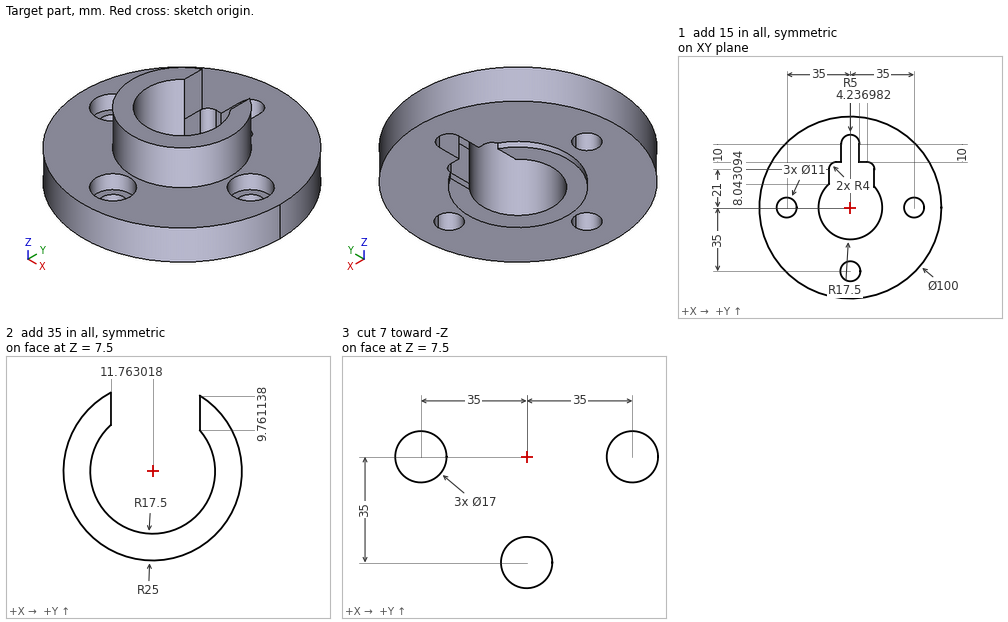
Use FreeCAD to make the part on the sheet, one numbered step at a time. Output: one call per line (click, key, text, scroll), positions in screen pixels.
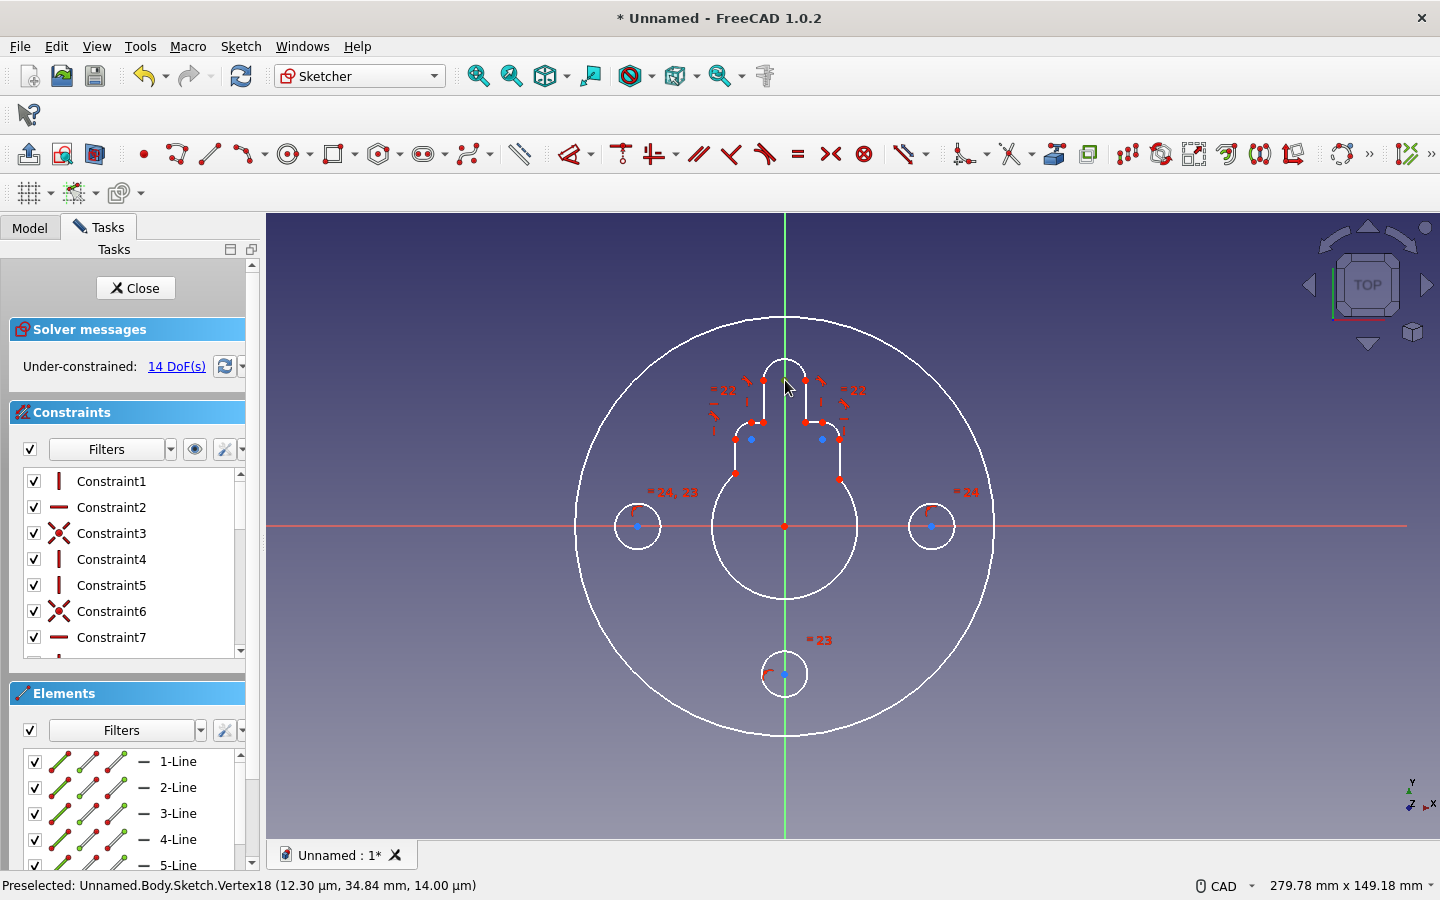
click(785, 770)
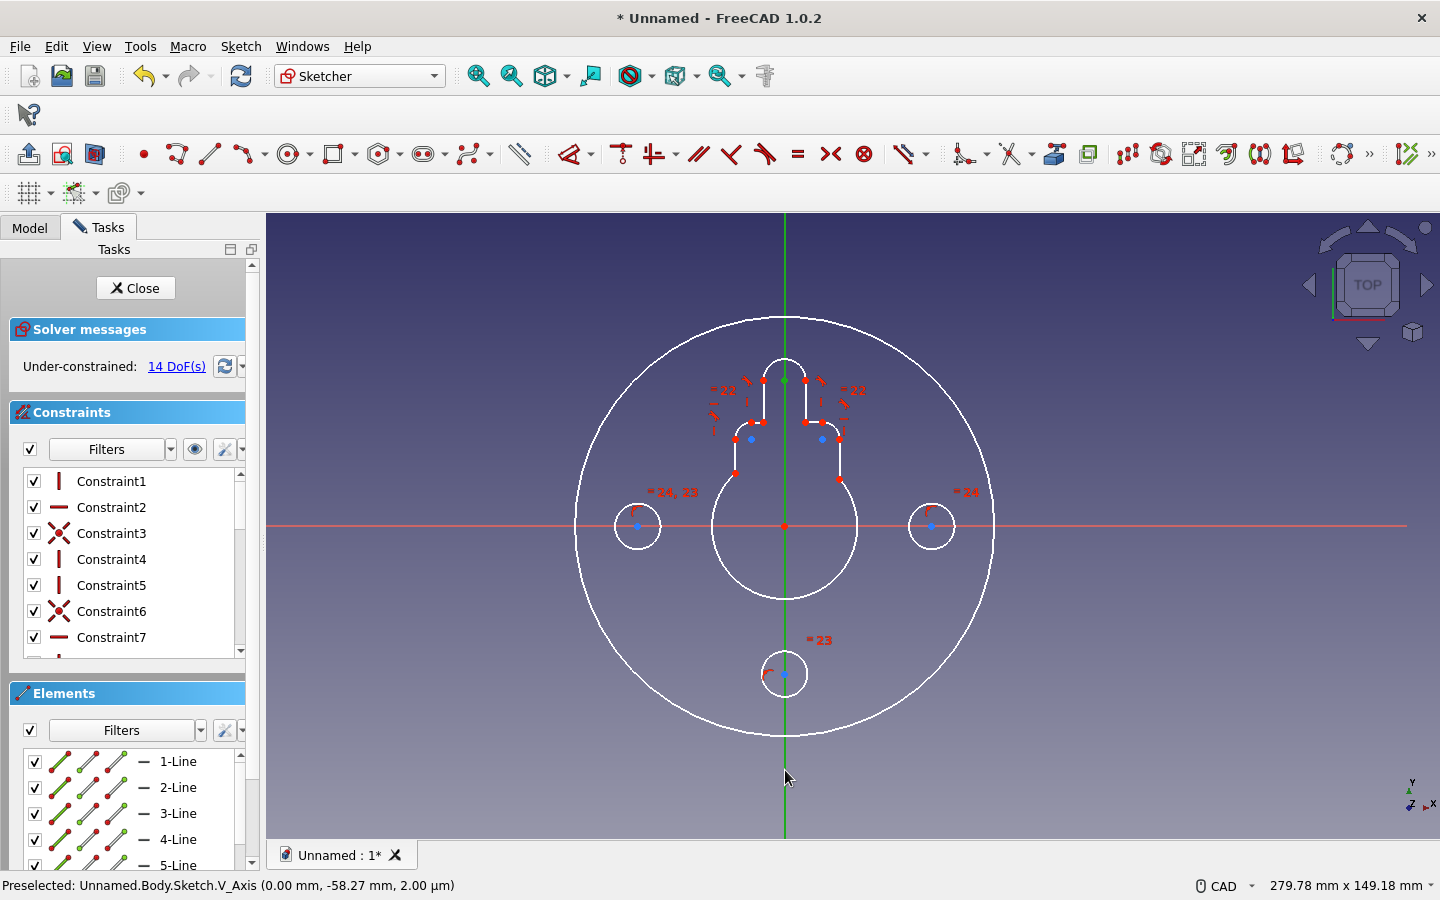
key(c)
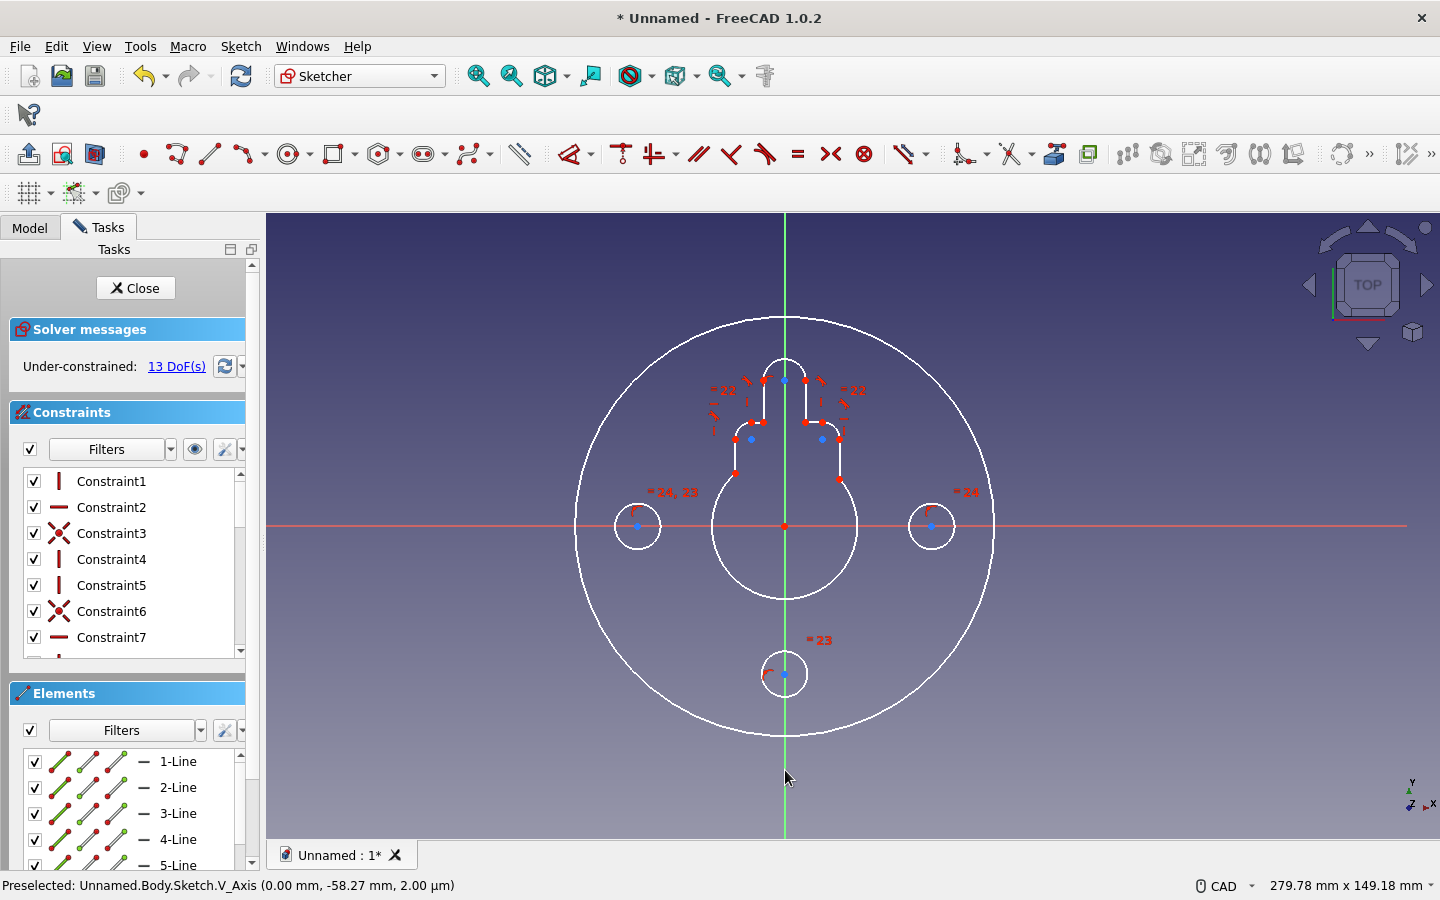
key(d)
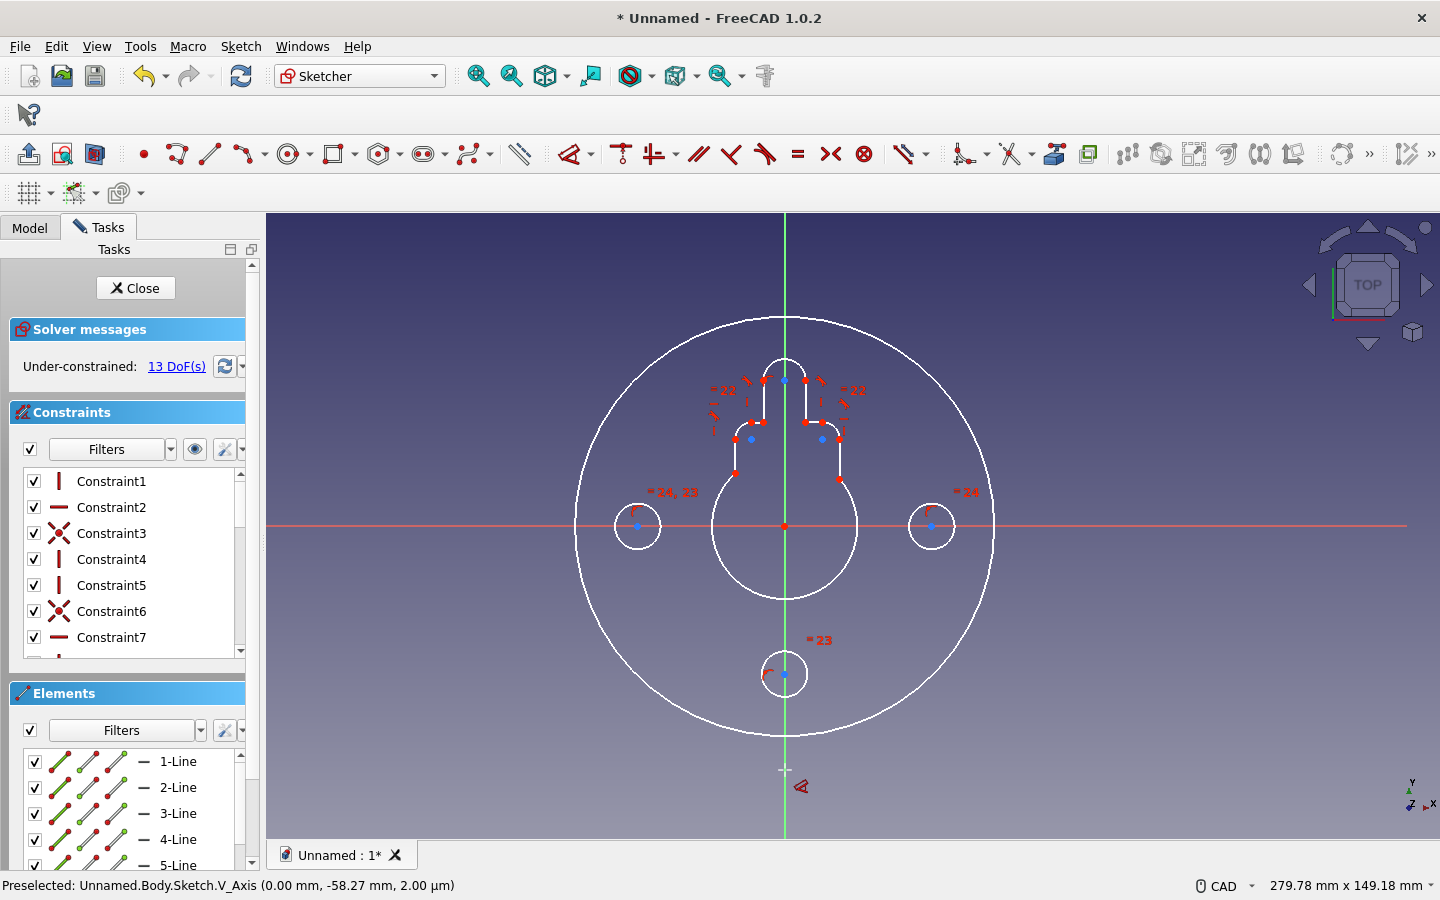
scroll(740, 427, up, 5)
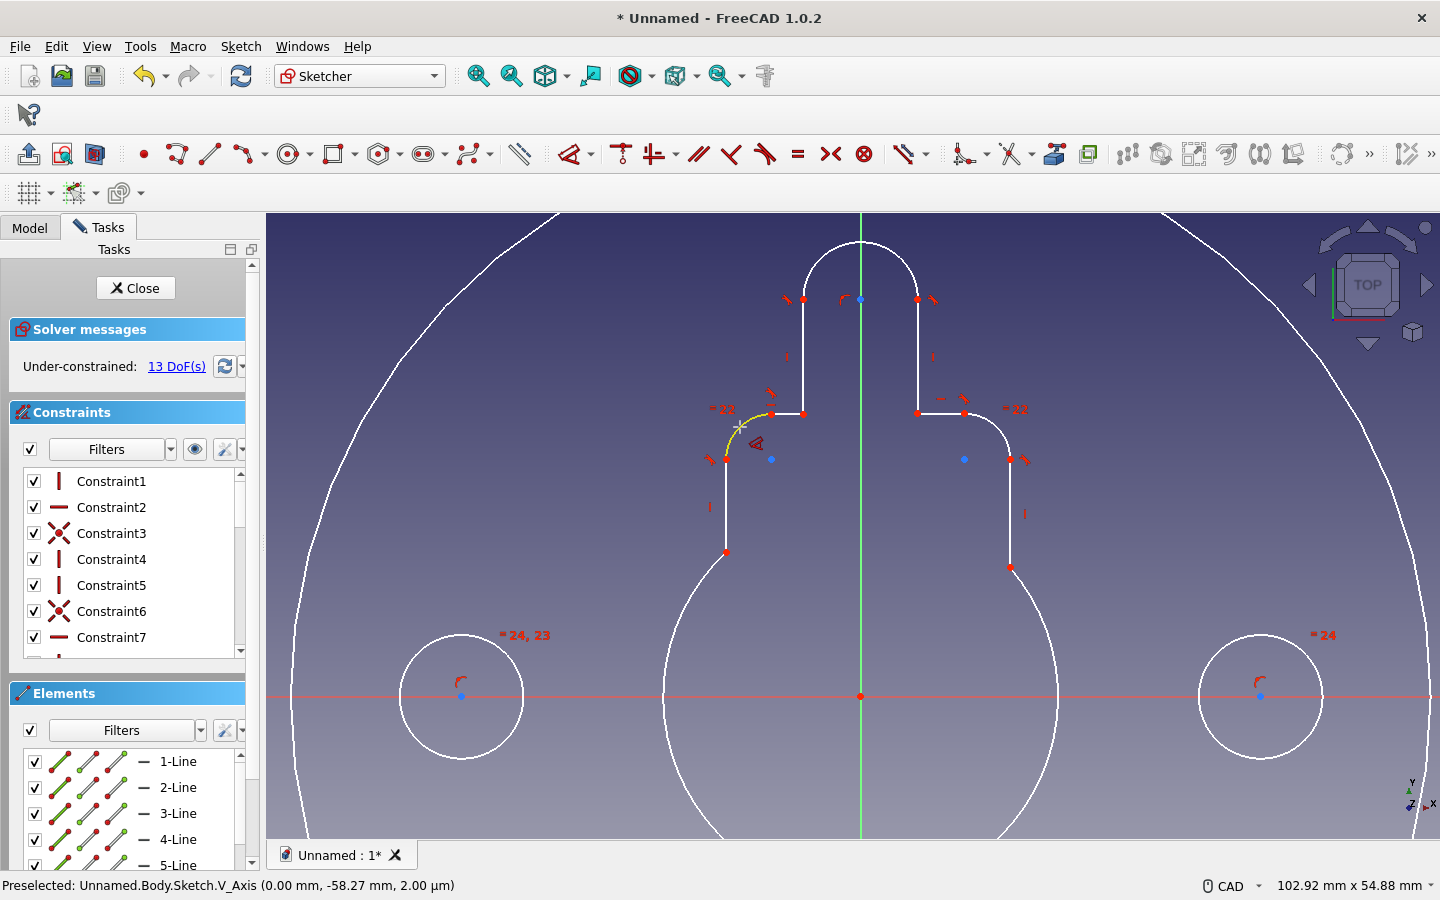
click(740, 428)
click(717, 405)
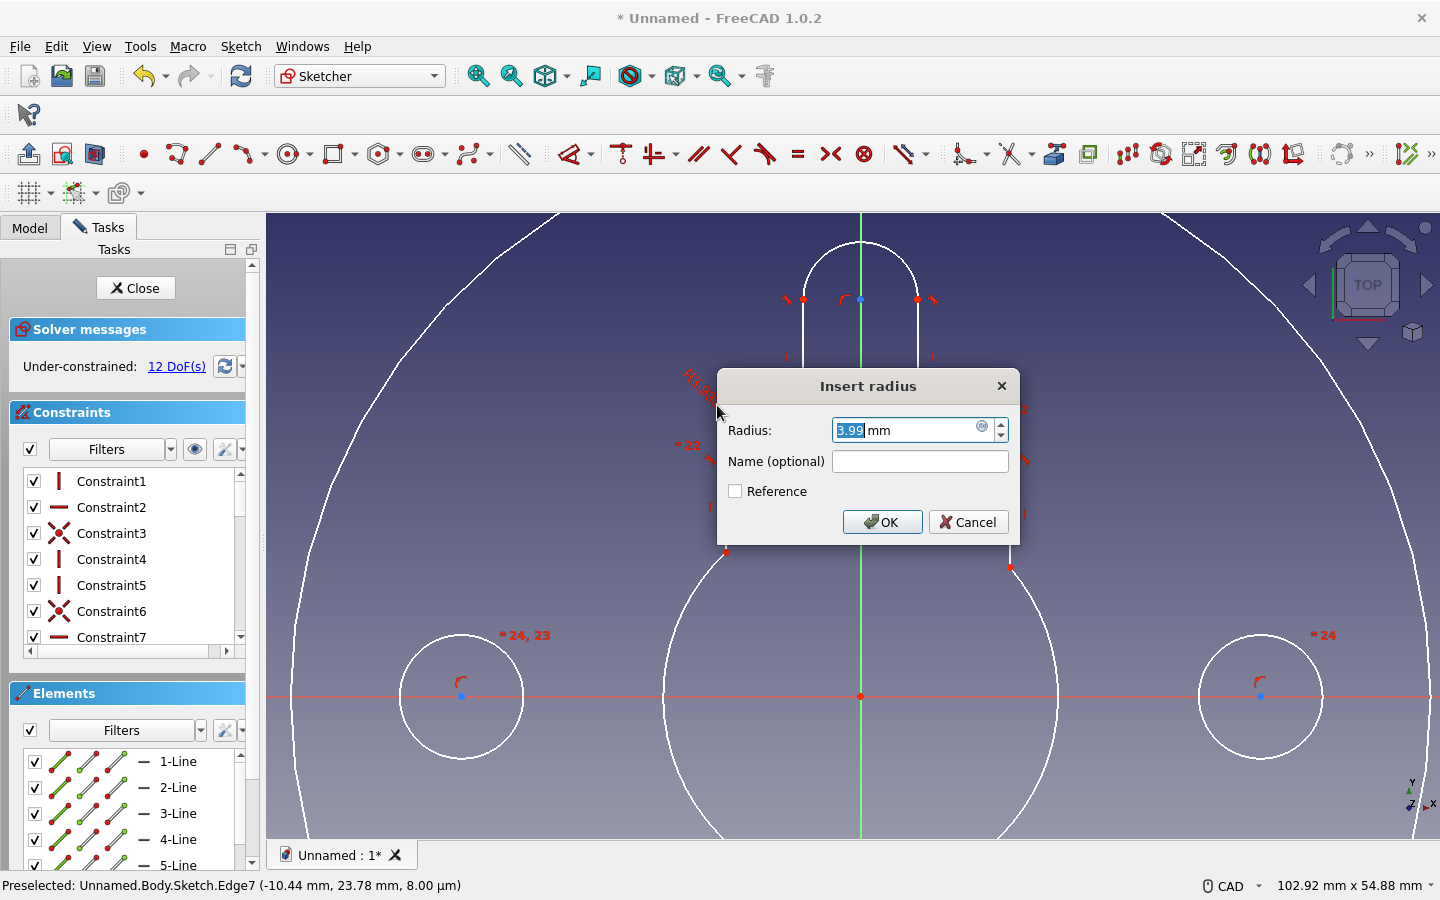
text(4)
key(Return)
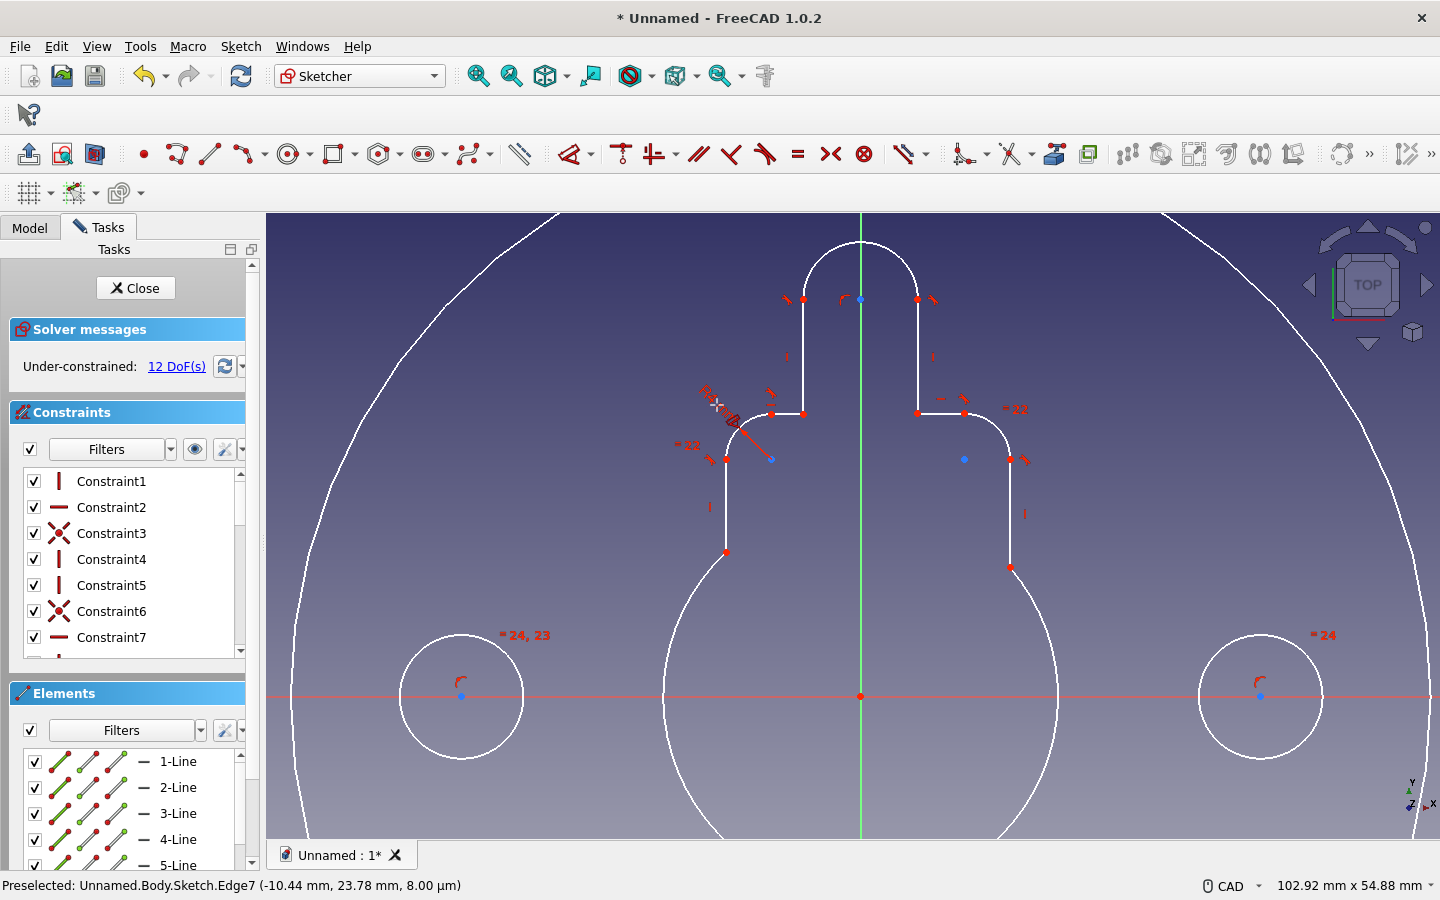
click(894, 253)
click(941, 261)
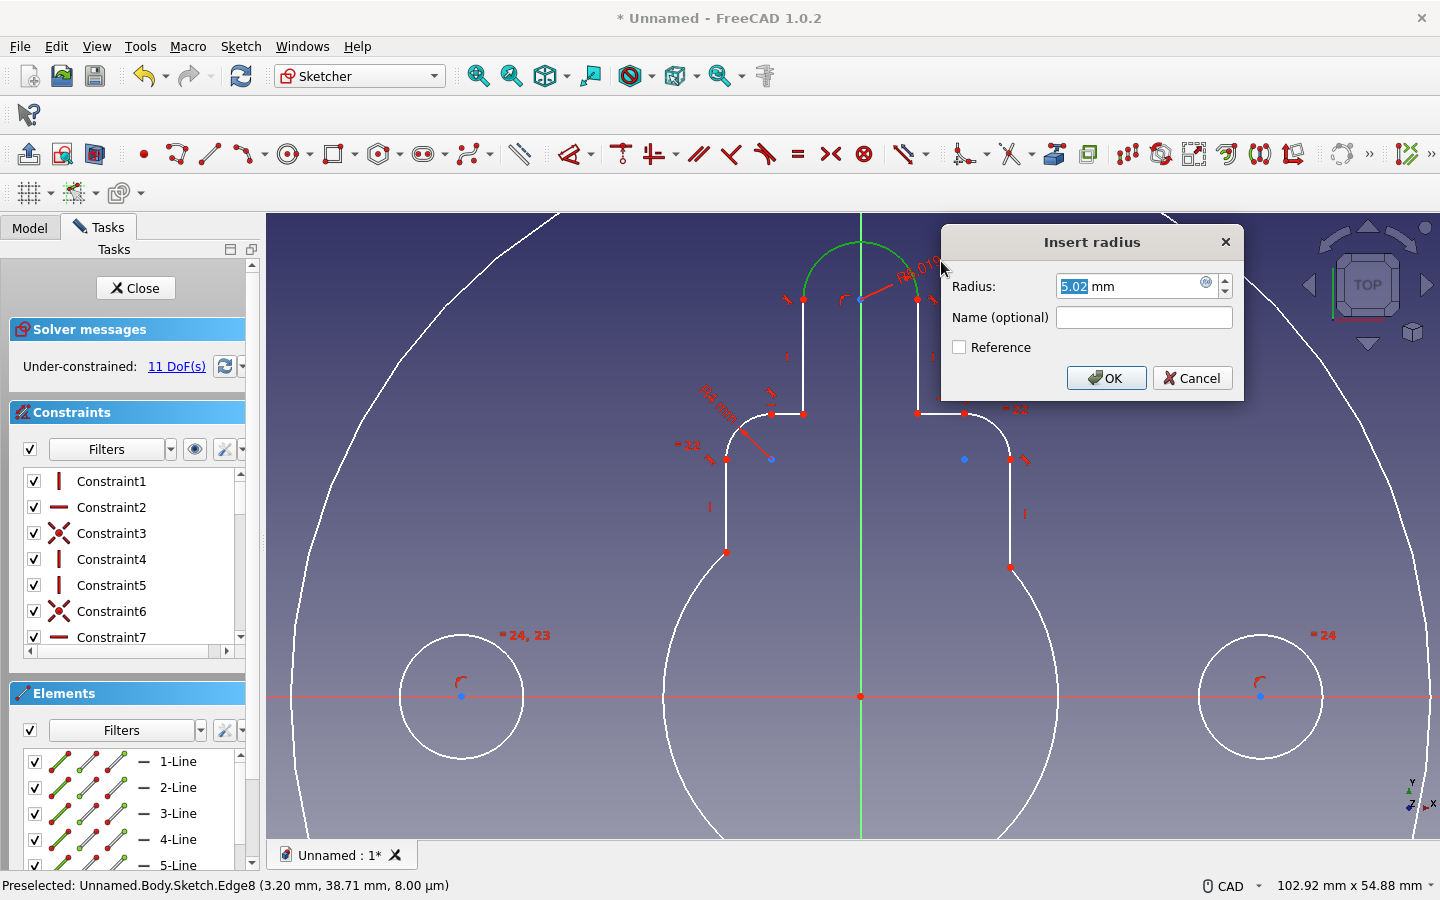
text(5)
key(Return)